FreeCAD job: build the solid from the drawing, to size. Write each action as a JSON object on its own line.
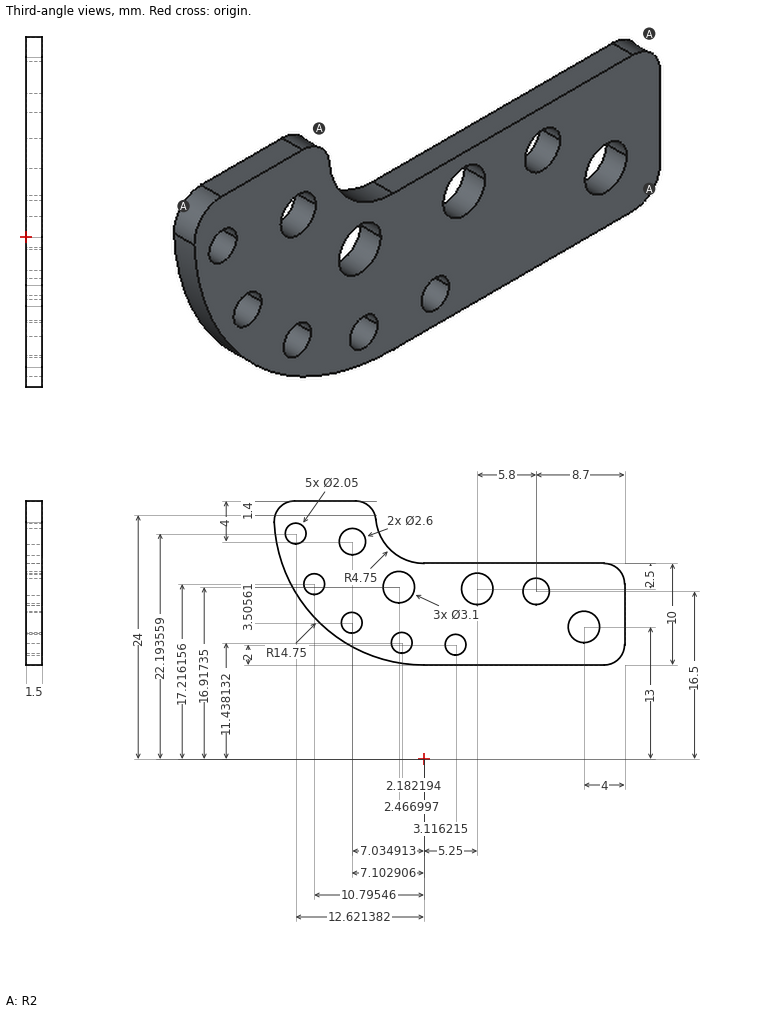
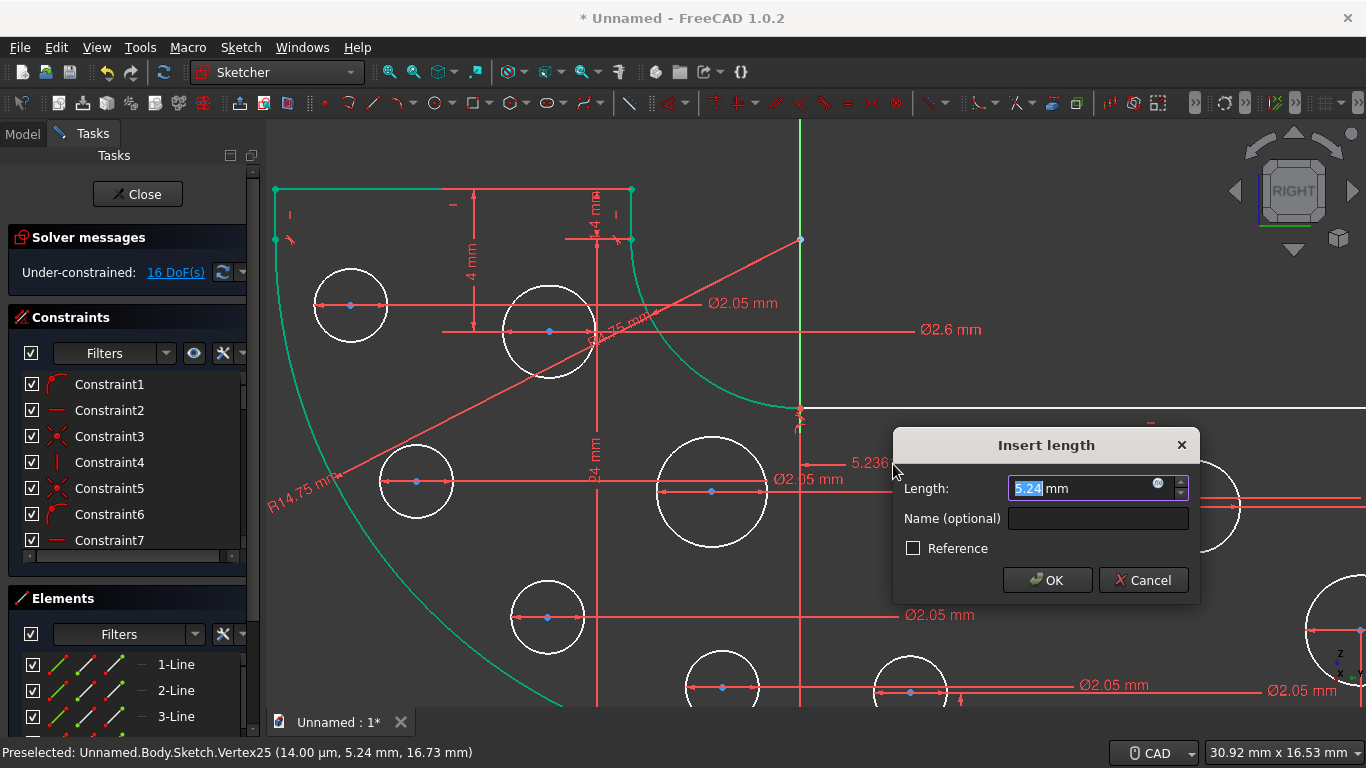
{"action": "type", "text": "5.25"}
{"action": "key", "text": "Return"}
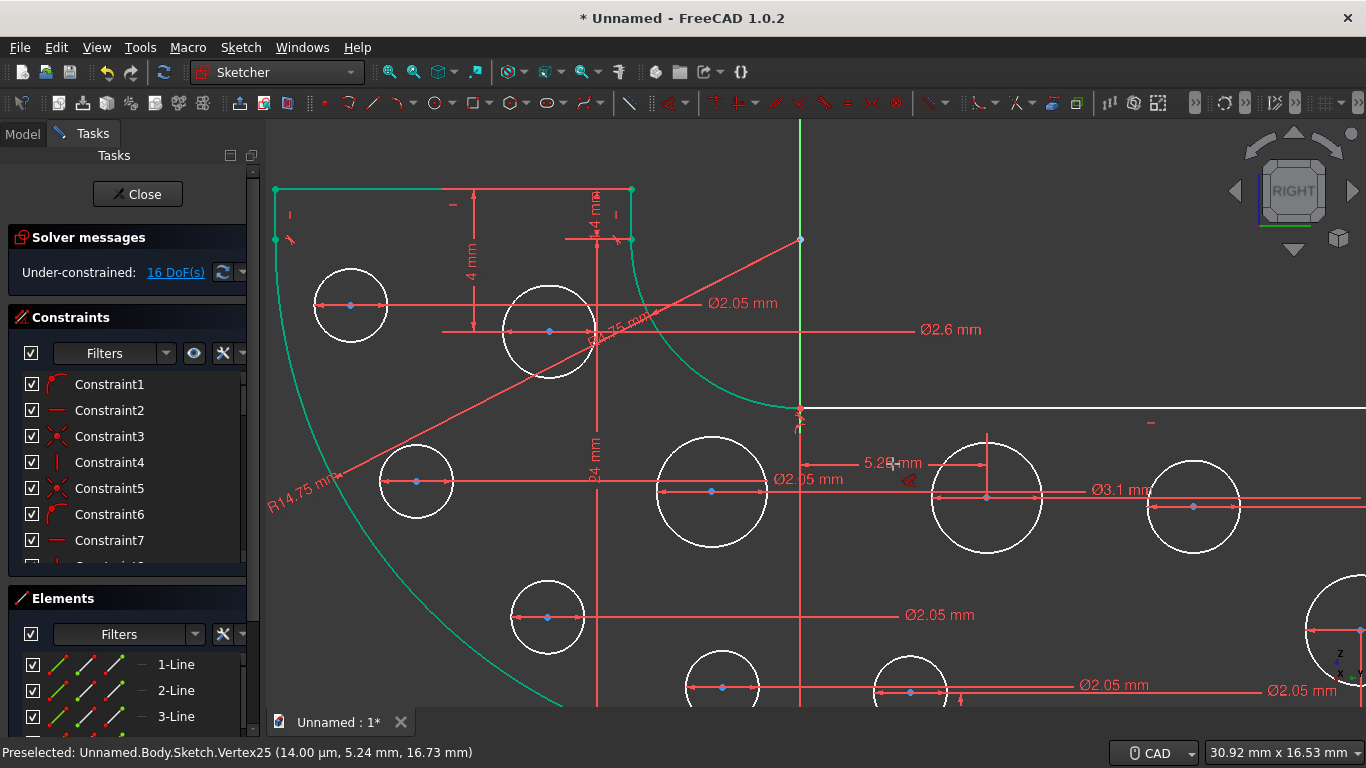
{"action": "left_click", "coordinate": [1194, 507]}
{"action": "left_click", "coordinate": [766, 593]}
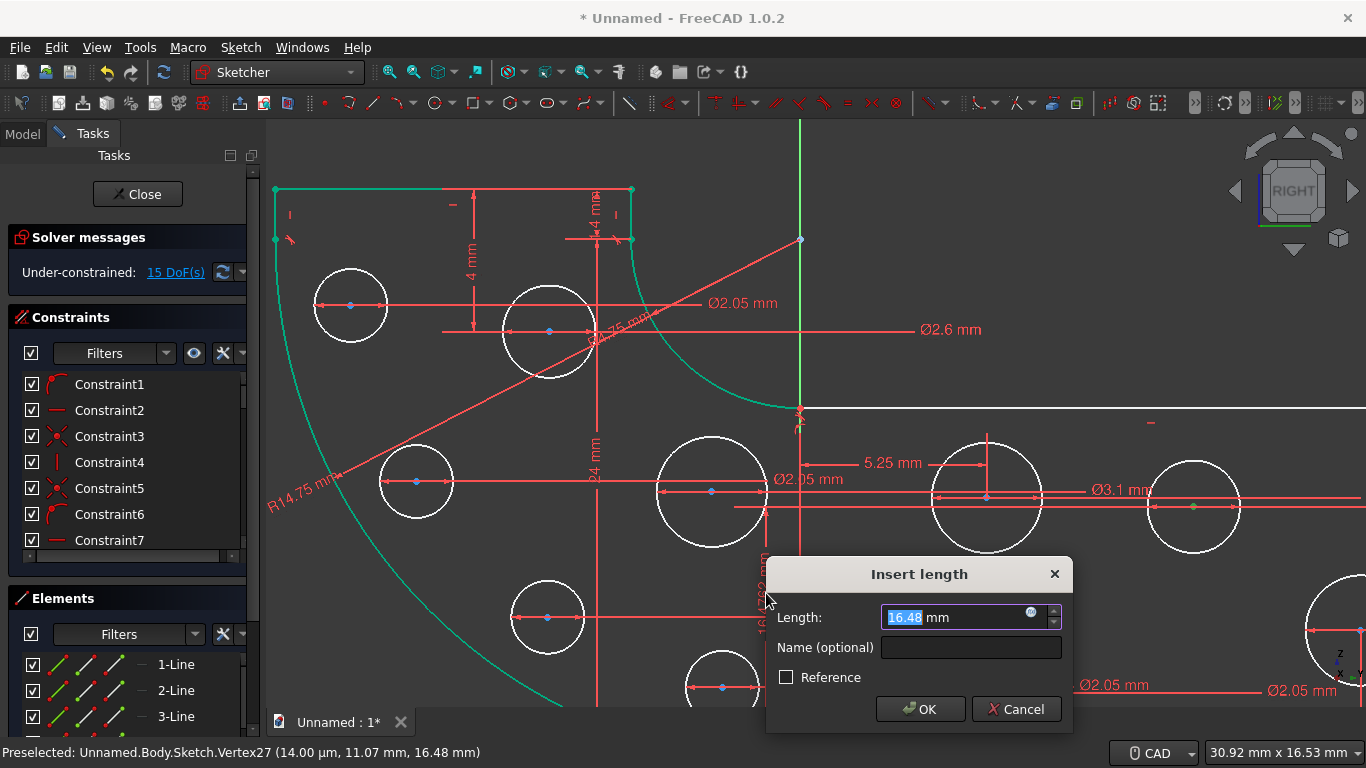
{"action": "type", "text": "16.5"}
{"action": "key", "text": "Return"}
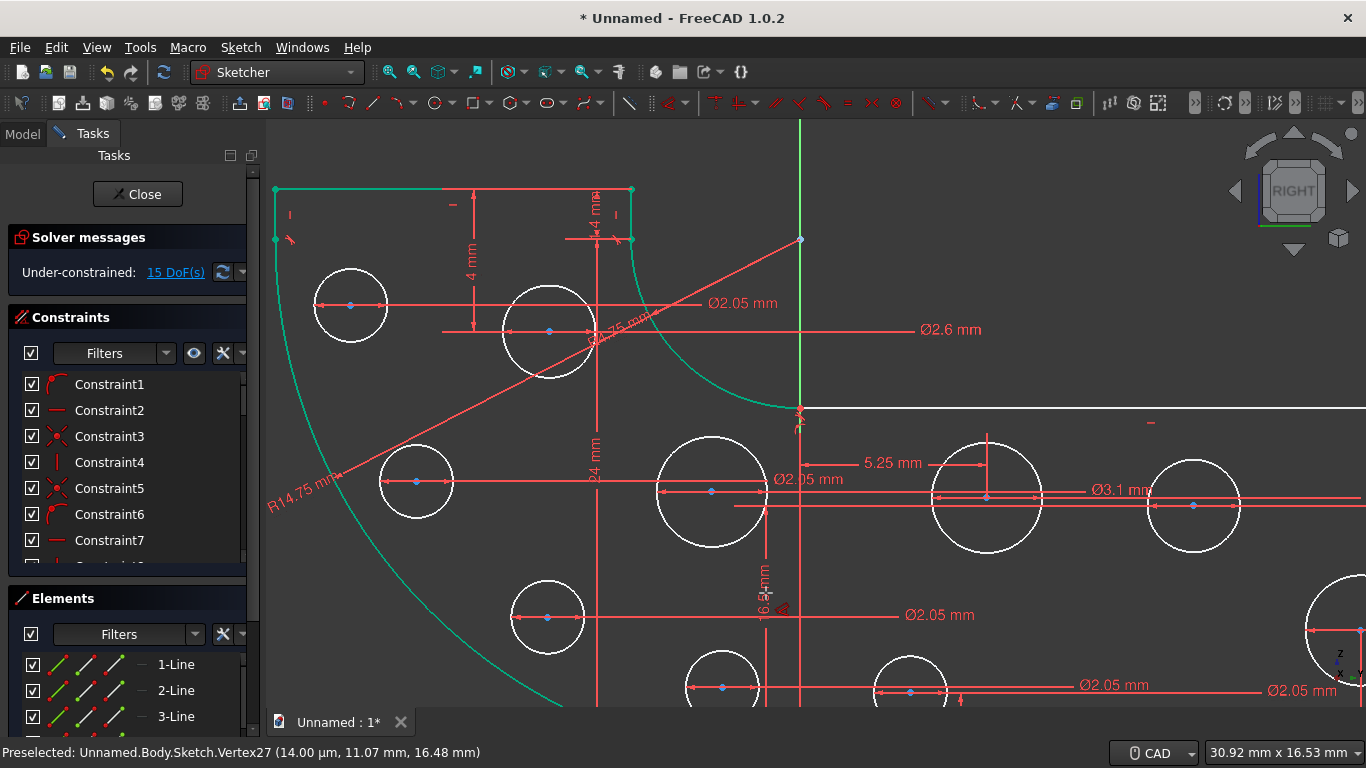
{"action": "left_click", "coordinate": [800, 408]}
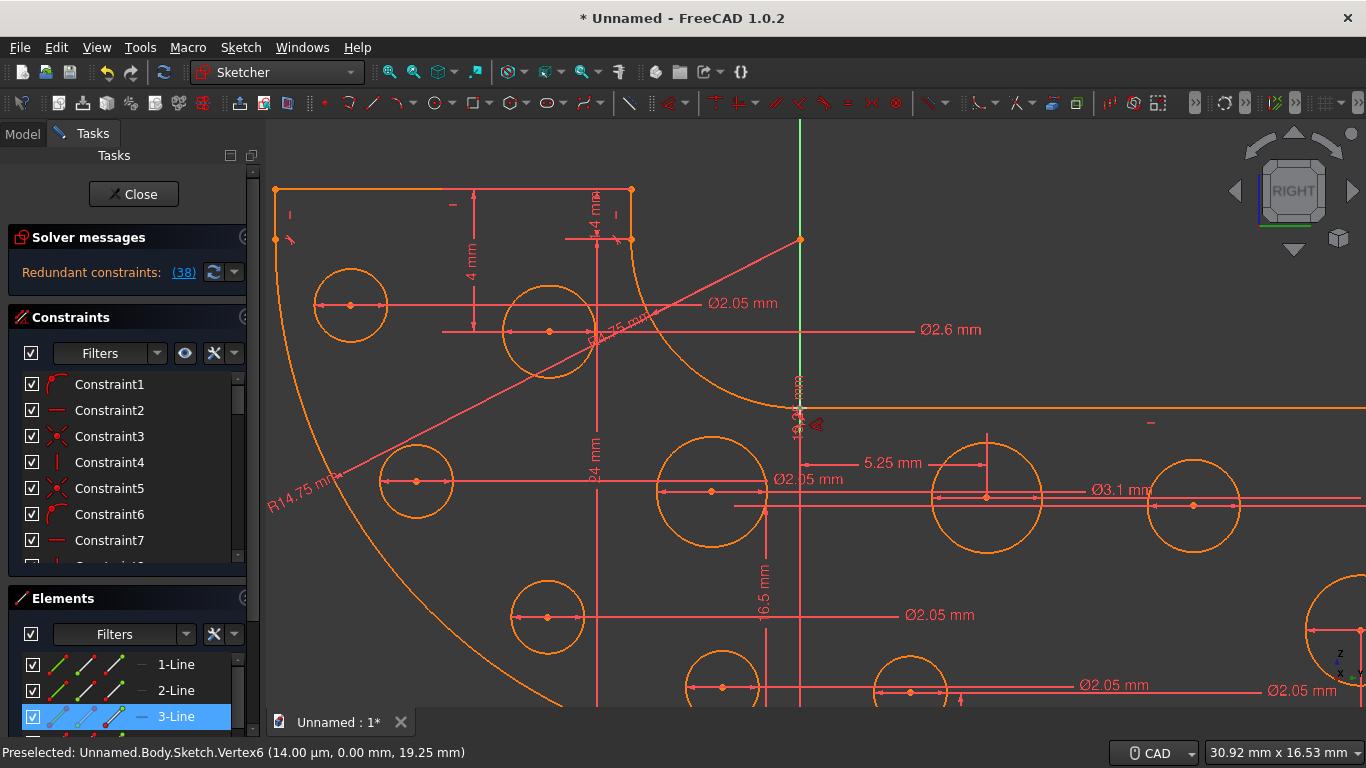
{"action": "left_click", "coordinate": [987, 498]}
{"action": "left_click", "coordinate": [1021, 432]}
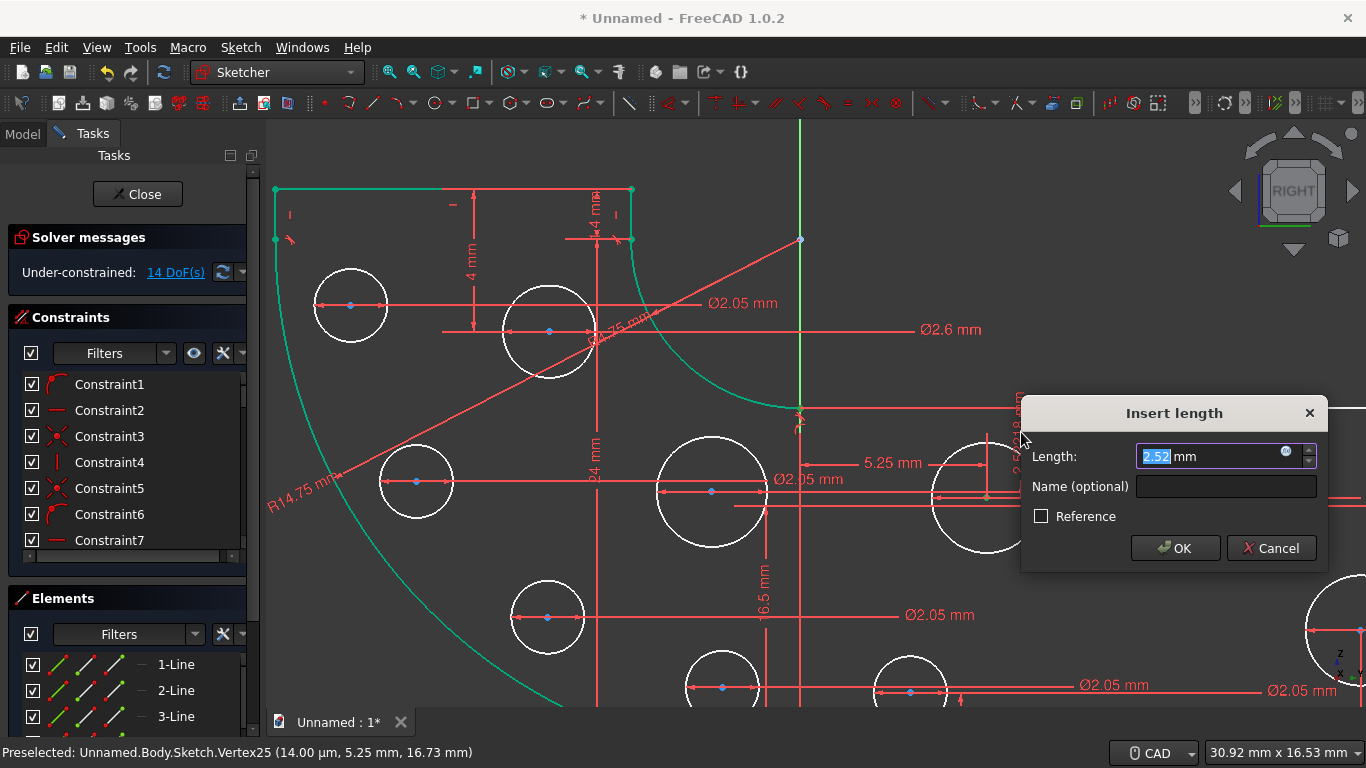
{"action": "type", "text": "2.5"}
{"action": "key", "text": "Return"}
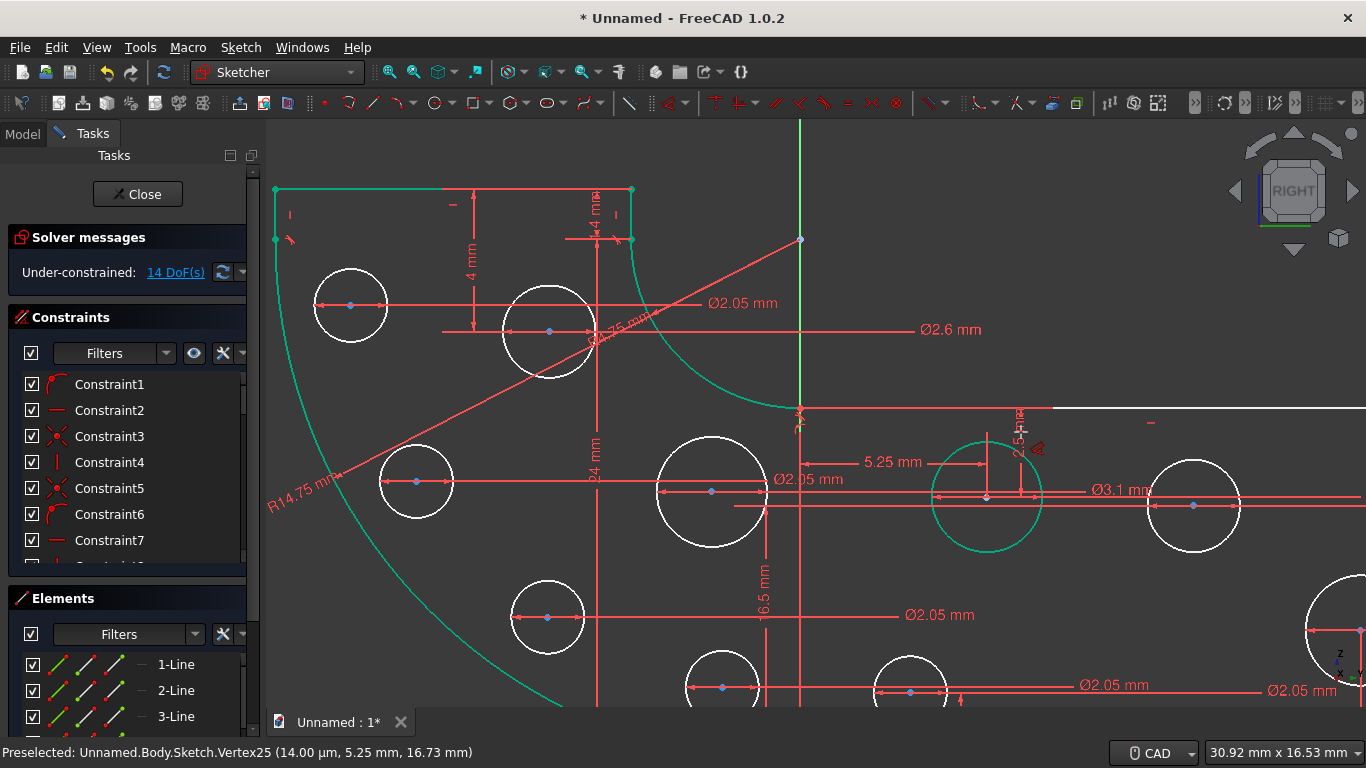
{"action": "left_click", "coordinate": [987, 497]}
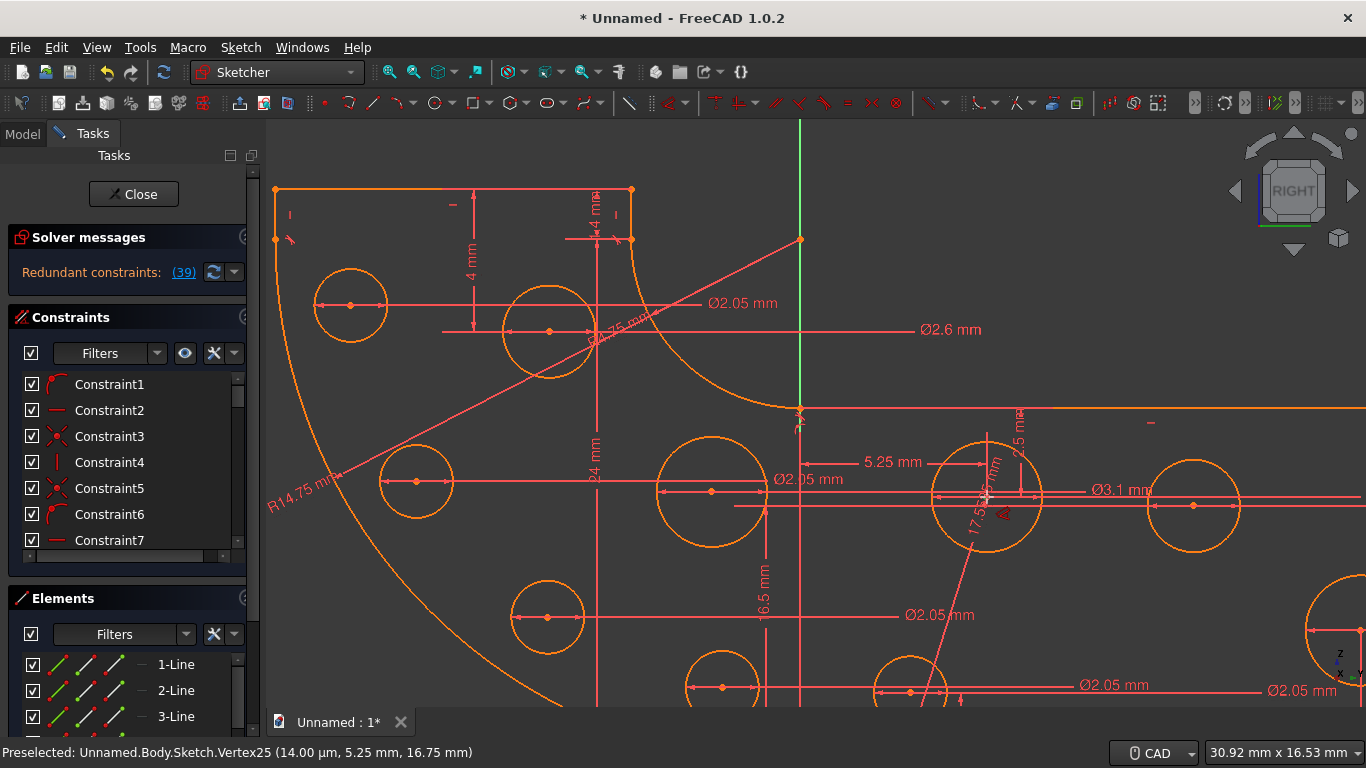
{"action": "left_click", "coordinate": [1194, 506]}
{"action": "left_click", "coordinate": [1090, 463]}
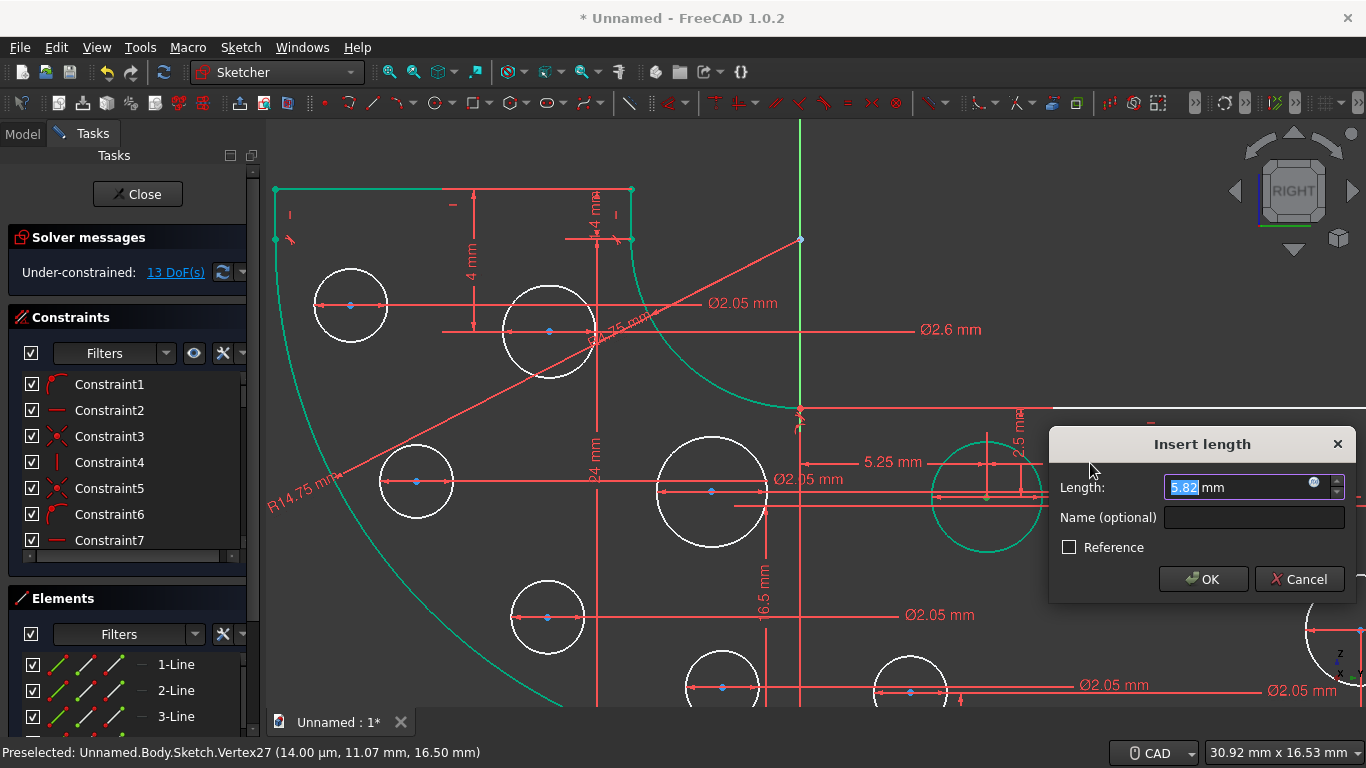
{"action": "type", "text": "5.8"}
{"action": "key", "text": "Return"}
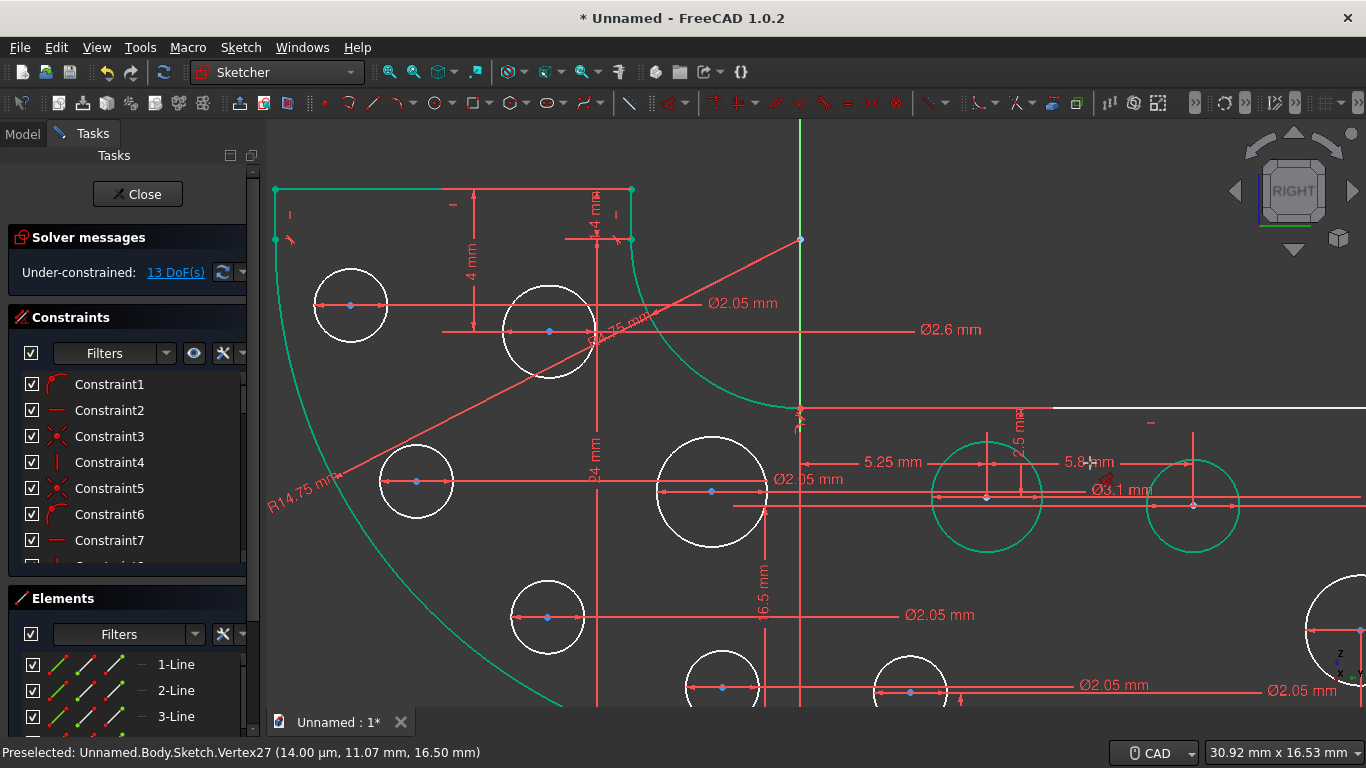
{"action": "scroll", "coordinate": [632, 227], "scroll_direction": "down", "scroll_amount": 4}